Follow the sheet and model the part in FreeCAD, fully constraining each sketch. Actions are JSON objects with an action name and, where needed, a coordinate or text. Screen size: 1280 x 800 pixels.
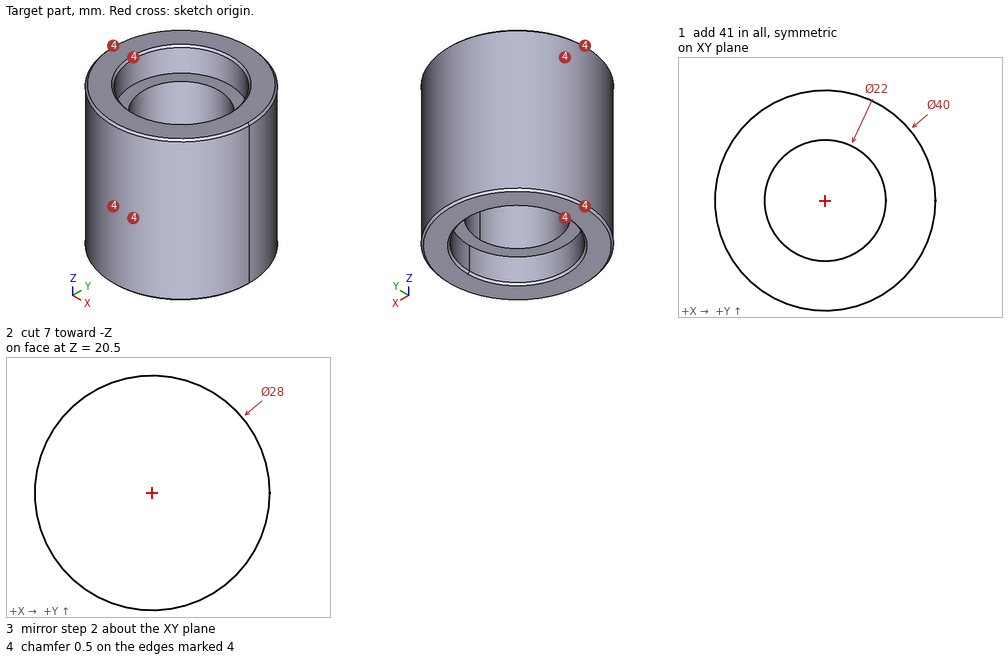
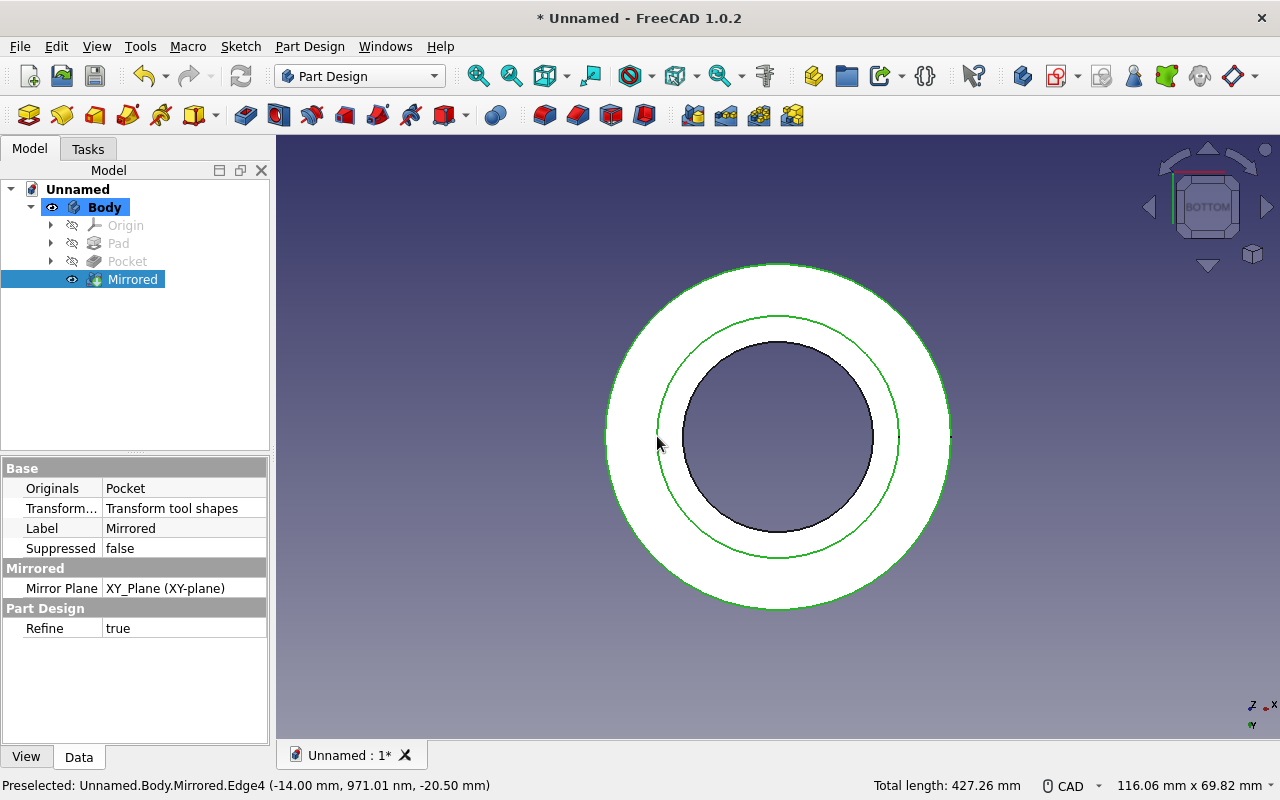
{"action": "left_click", "coordinate": [578, 116]}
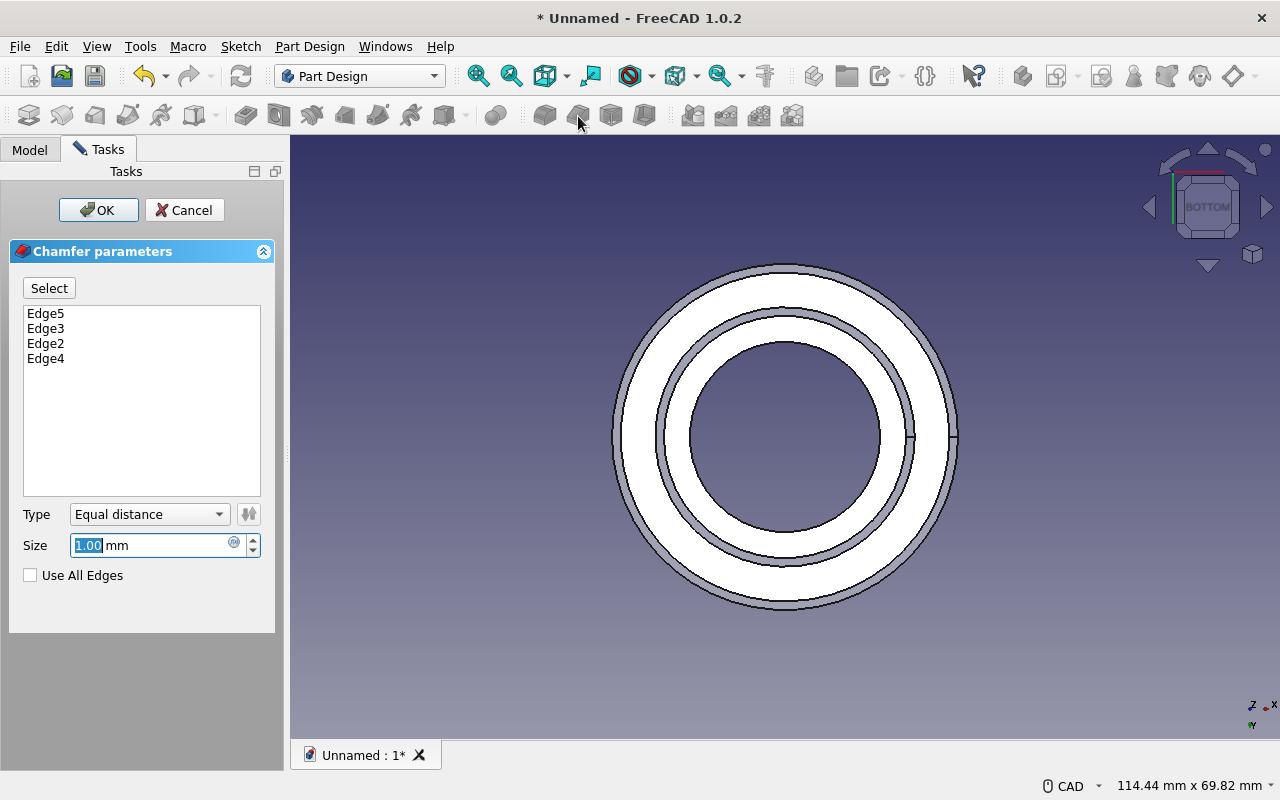
{"action": "type", "text": "0.5"}
{"action": "key", "text": "Tab"}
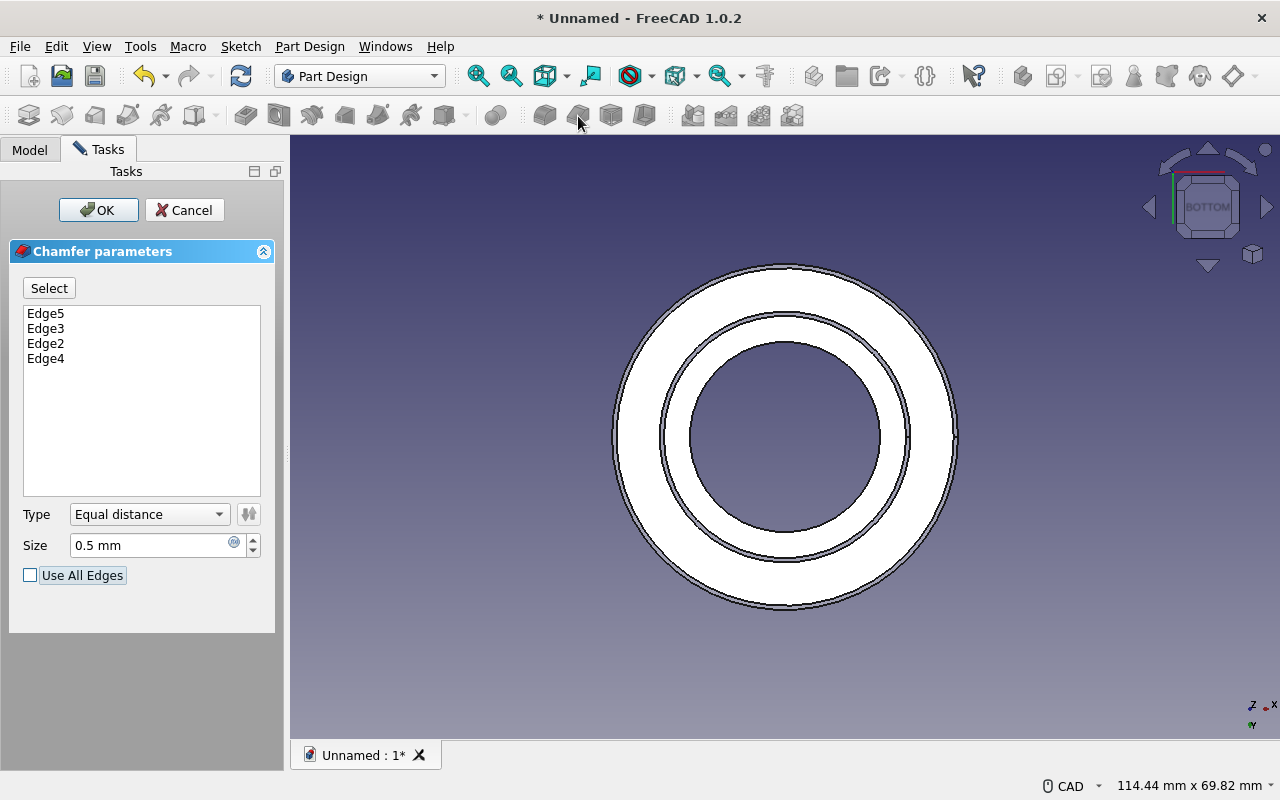
{"action": "left_click", "coordinate": [99, 210]}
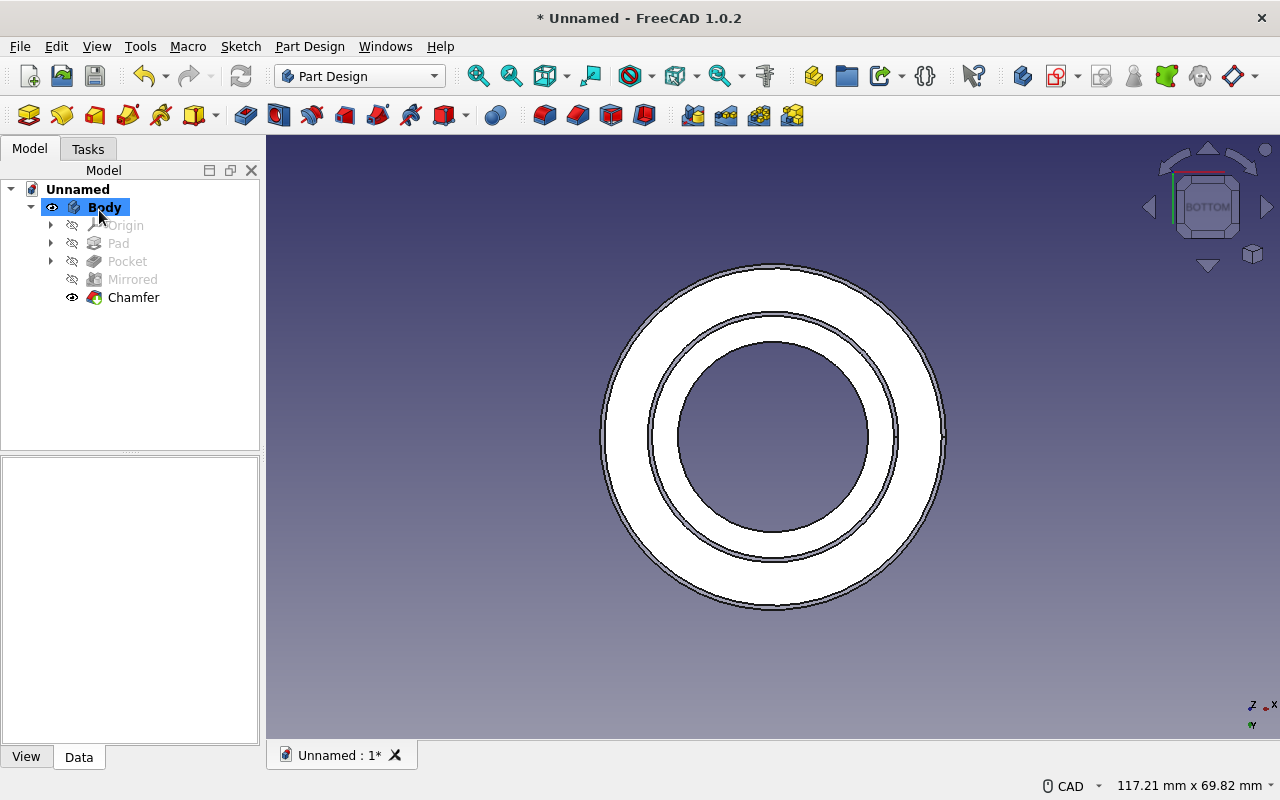
{"action": "key", "text": "0"}